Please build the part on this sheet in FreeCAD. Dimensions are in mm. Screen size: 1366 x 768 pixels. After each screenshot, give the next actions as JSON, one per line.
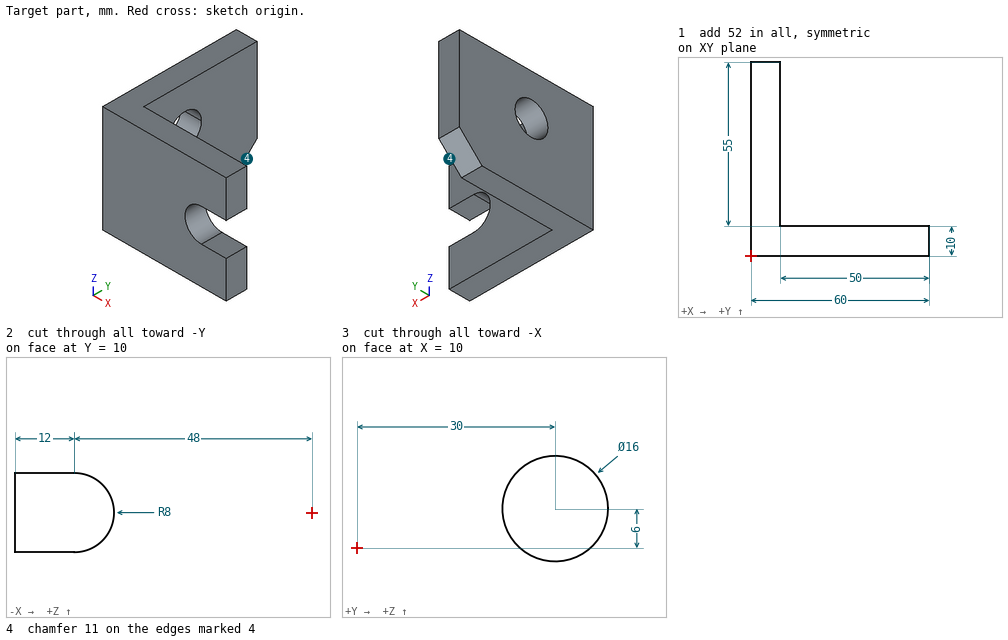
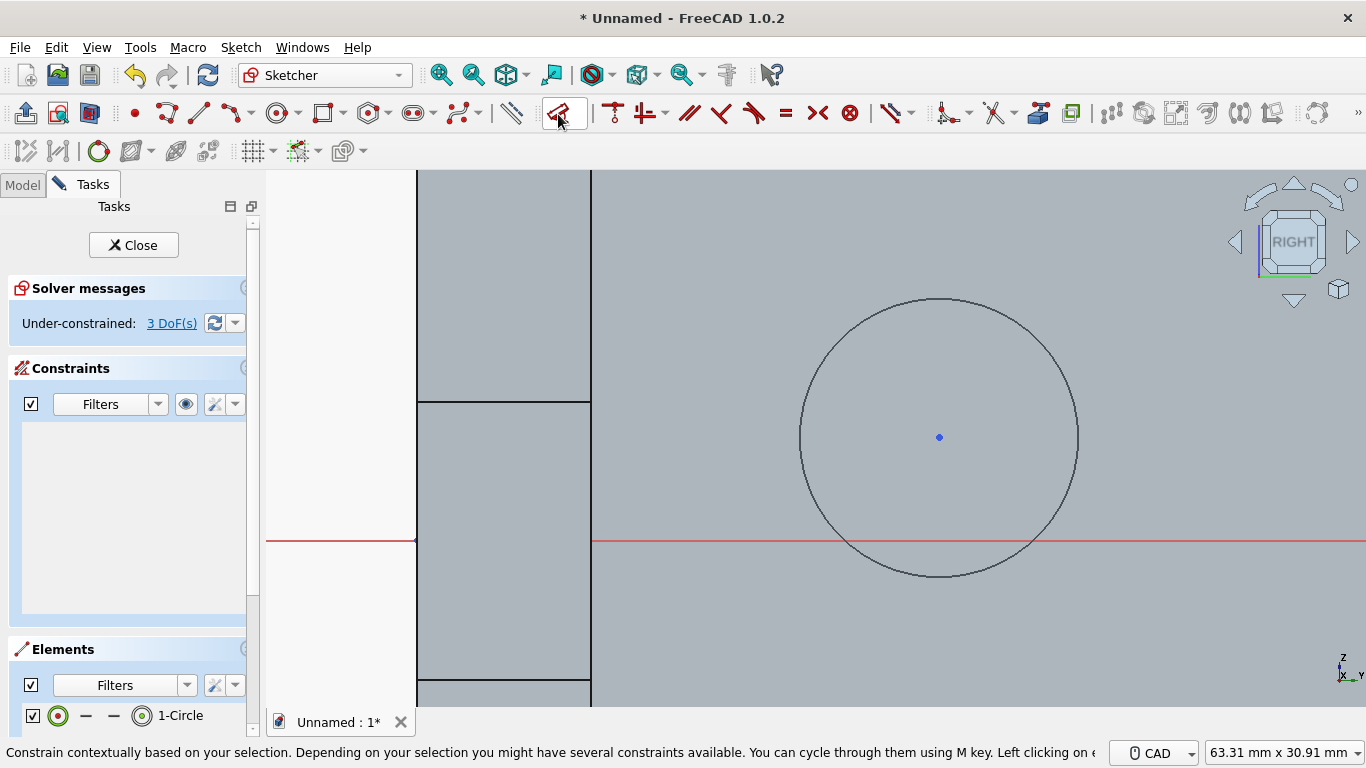
{"action": "left_click", "coordinate": [1037, 339]}
{"action": "left_click", "coordinate": [1060, 316]}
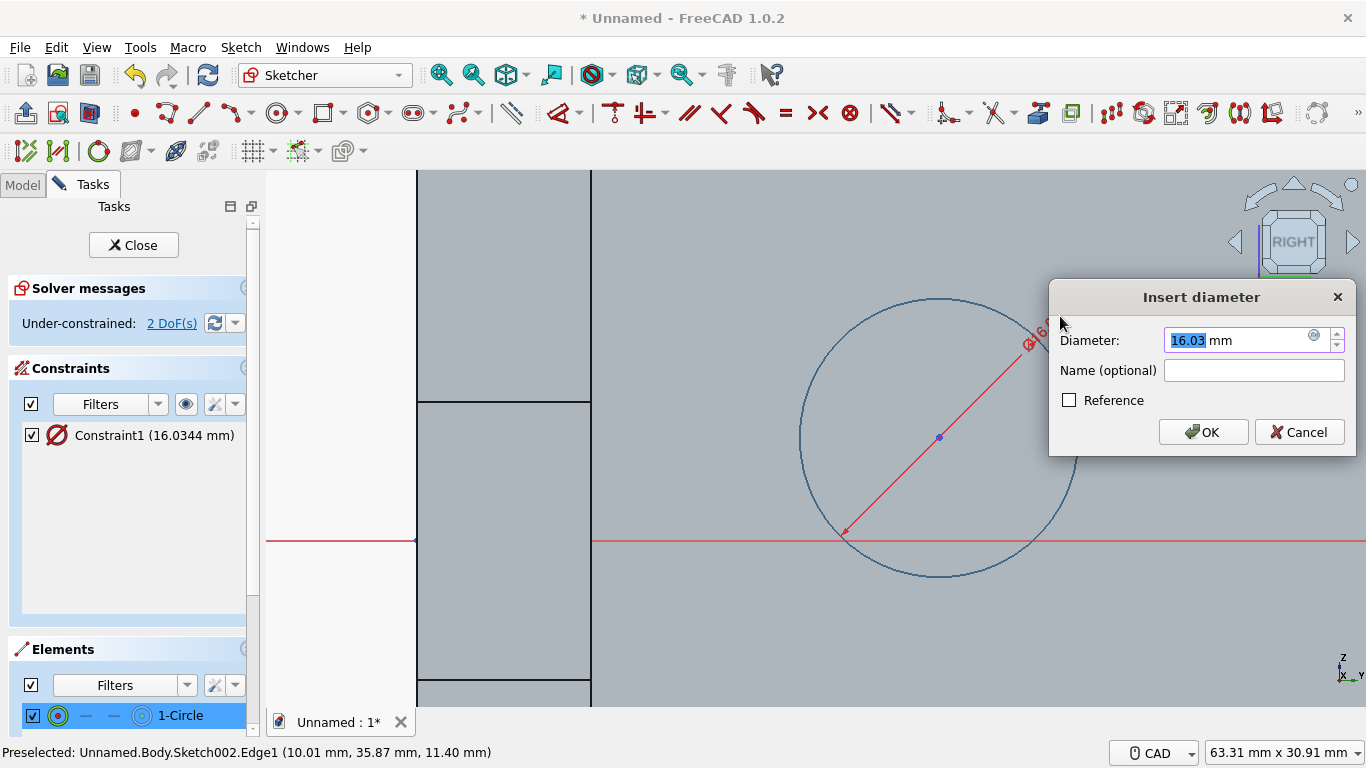
{"action": "type", "text": "16"}
{"action": "key", "text": "Return"}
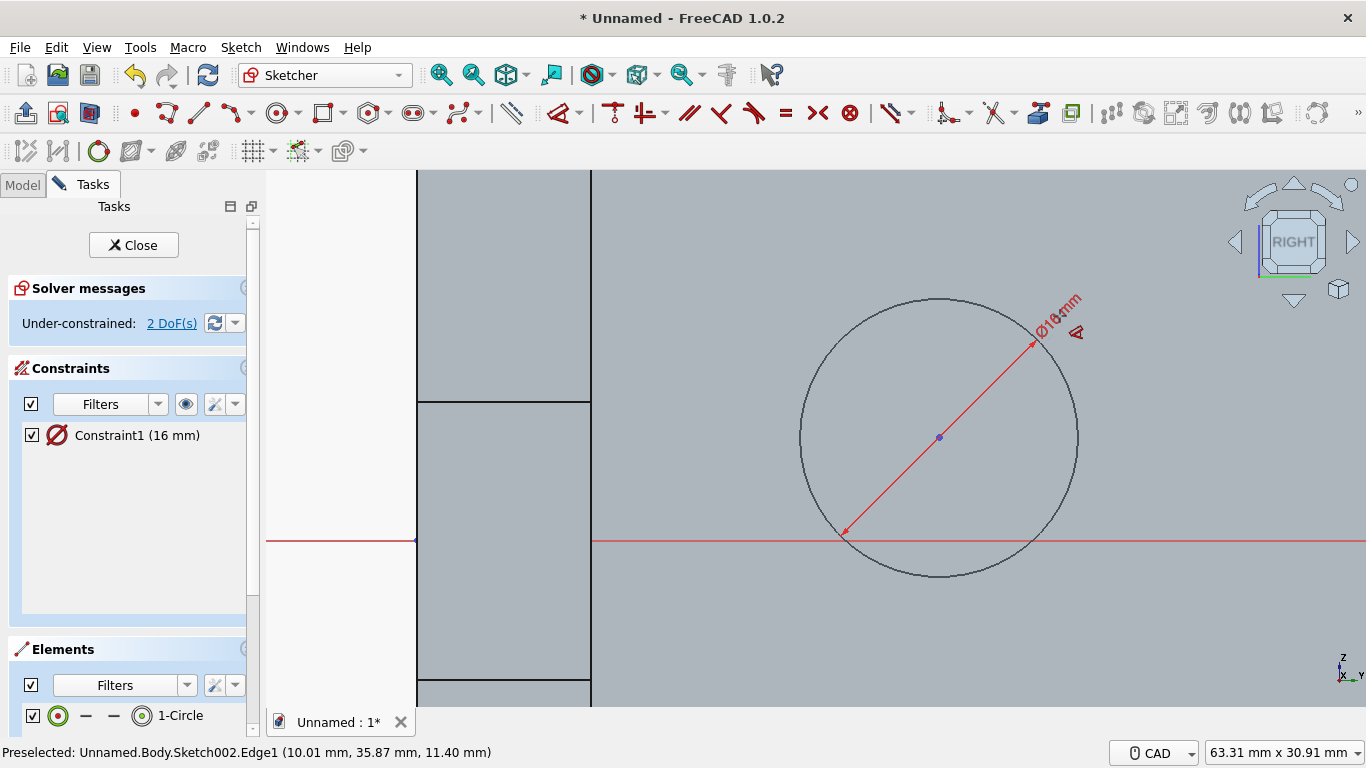
{"action": "left_click", "coordinate": [939, 438]}
{"action": "left_click", "coordinate": [383, 489]}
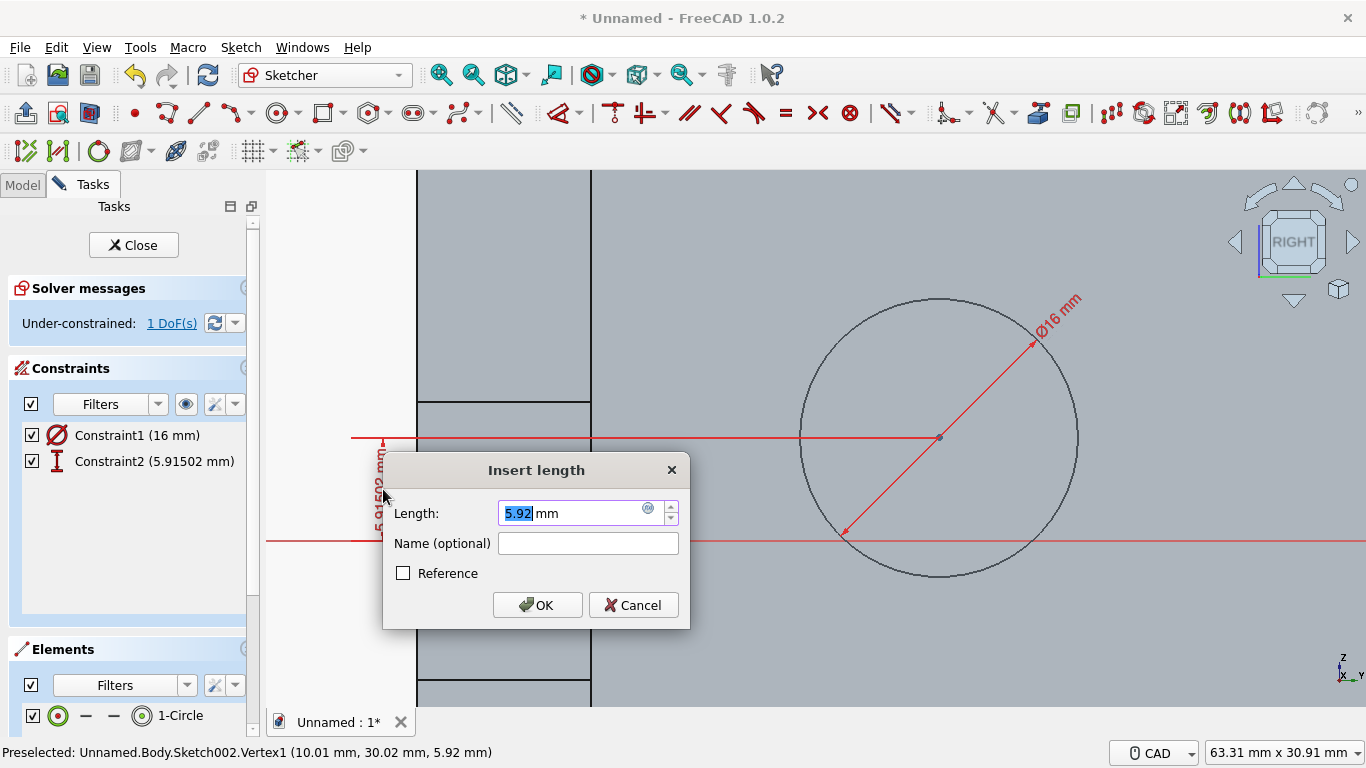
{"action": "type", "text": "6"}
{"action": "key", "text": "Return"}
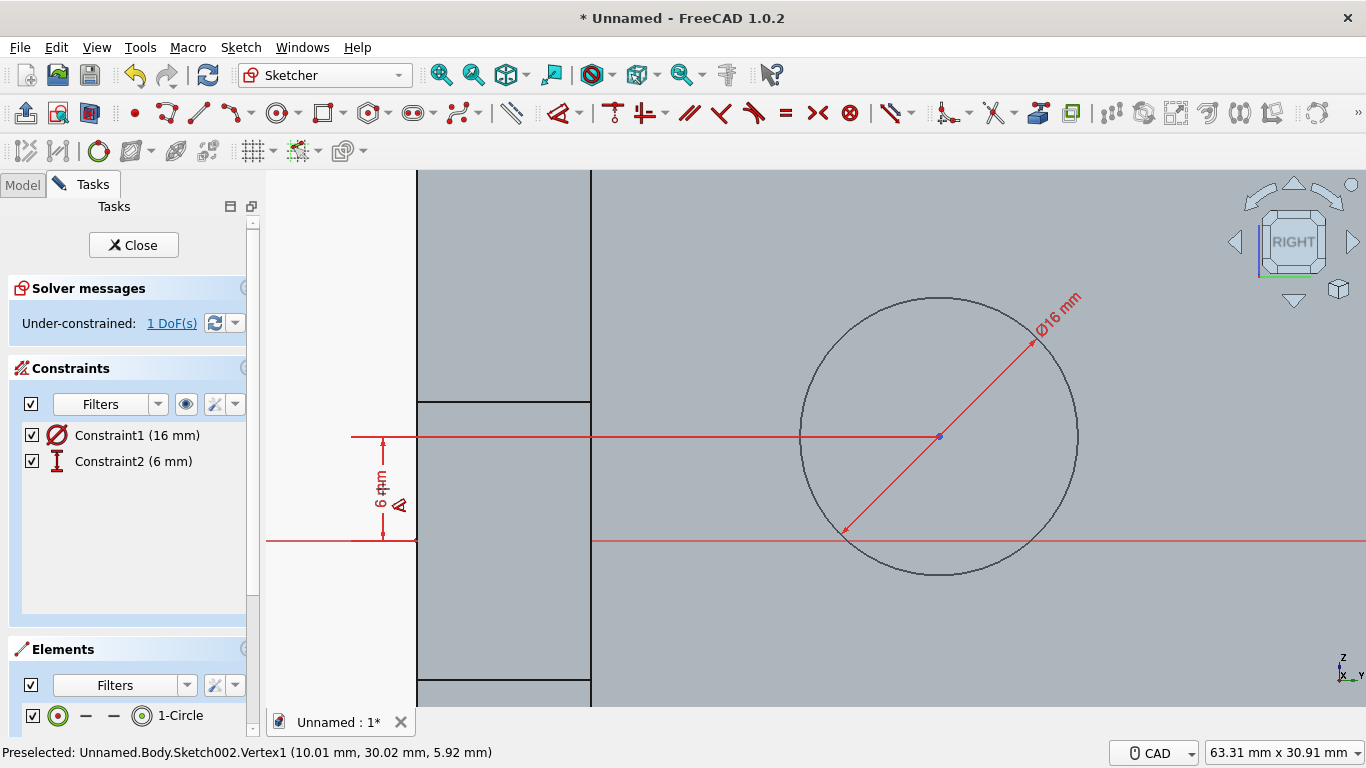
{"action": "left_click", "coordinate": [939, 437]}
{"action": "left_click", "coordinate": [678, 575]}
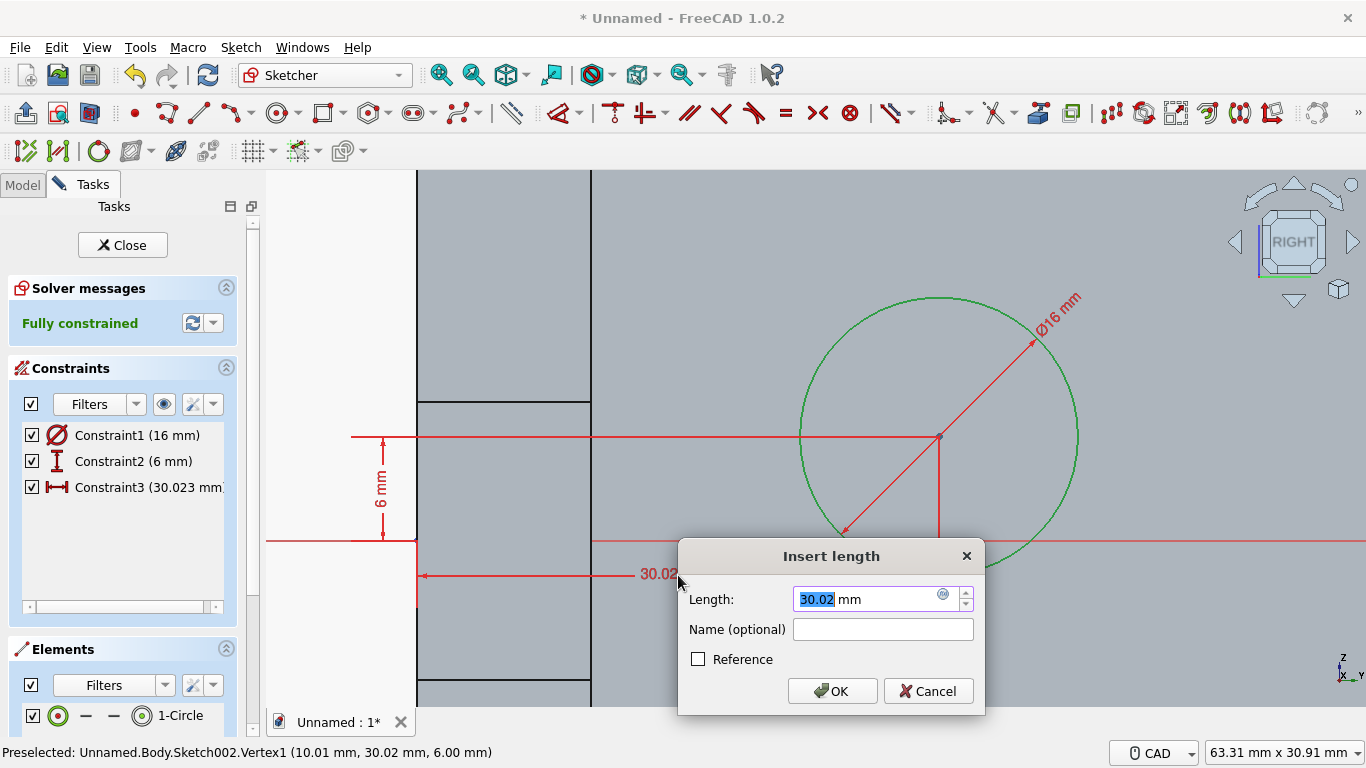
{"action": "type", "text": "30"}
{"action": "key", "text": "Return"}
{"action": "key", "text": "Escape"}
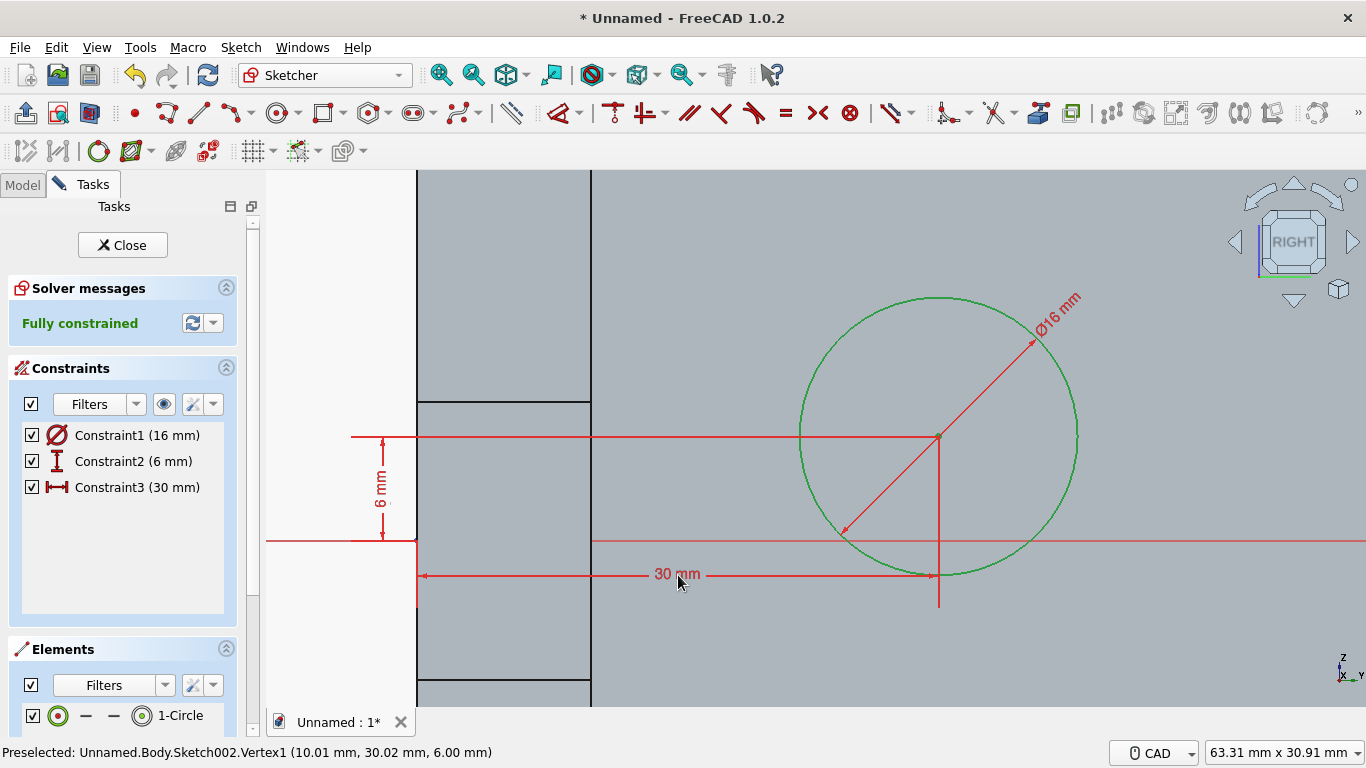
{"action": "left_click", "coordinate": [123, 245]}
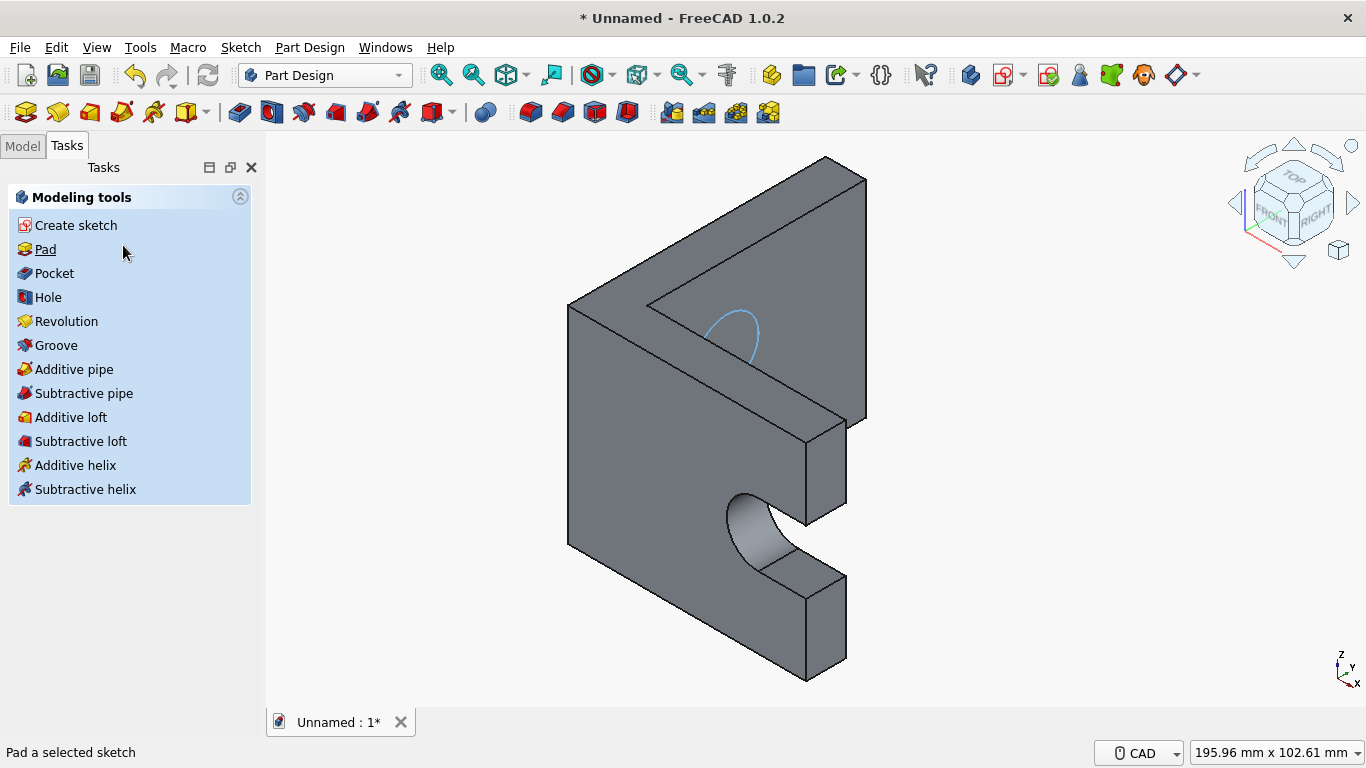
{"action": "left_click", "coordinate": [240, 112]}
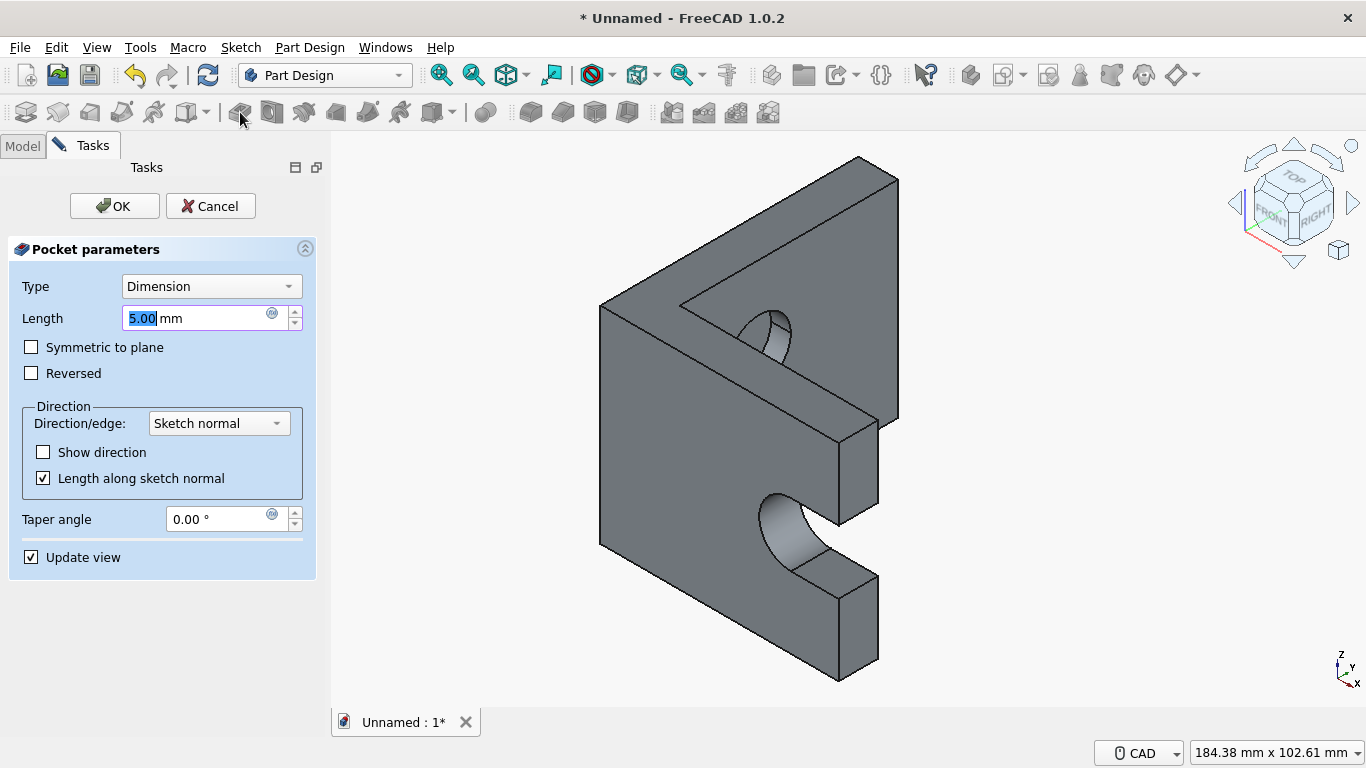
{"action": "left_click", "coordinate": [212, 286]}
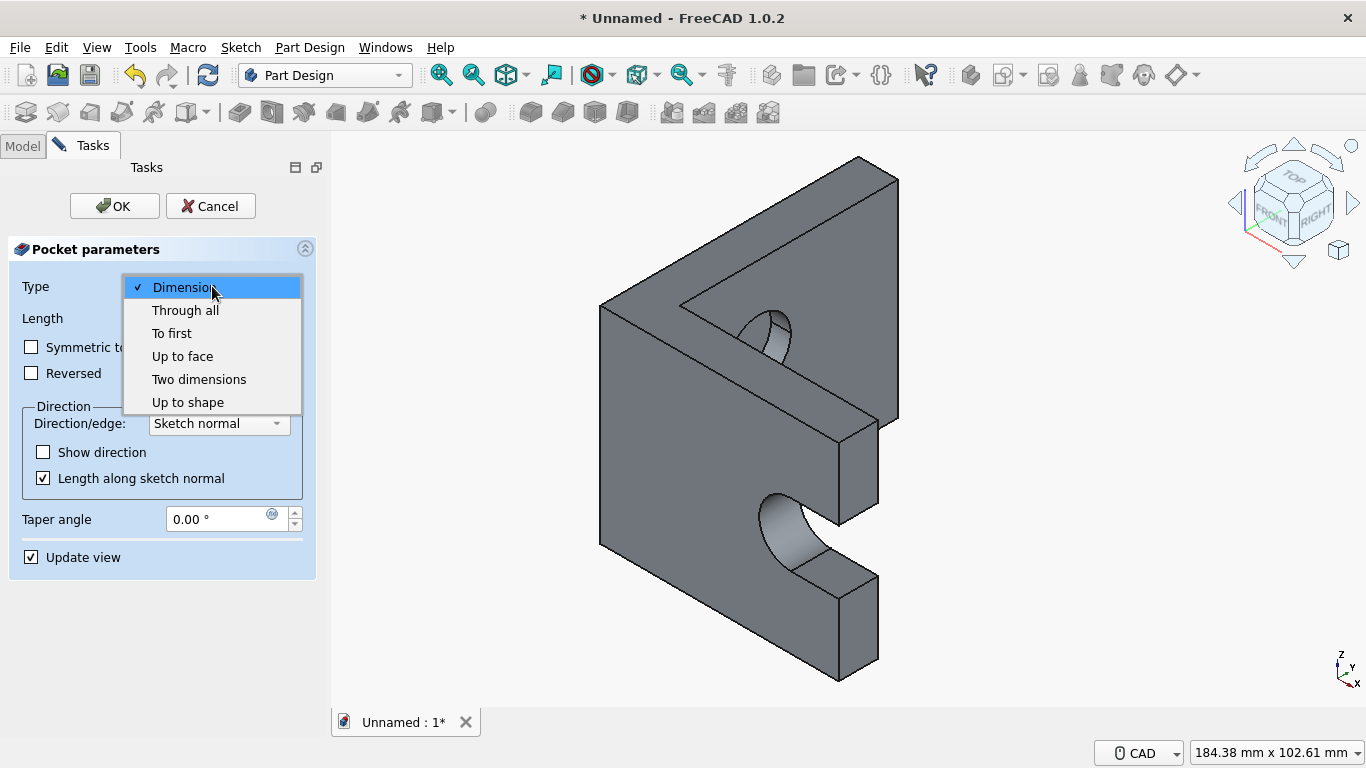
{"action": "left_click", "coordinate": [212, 310]}